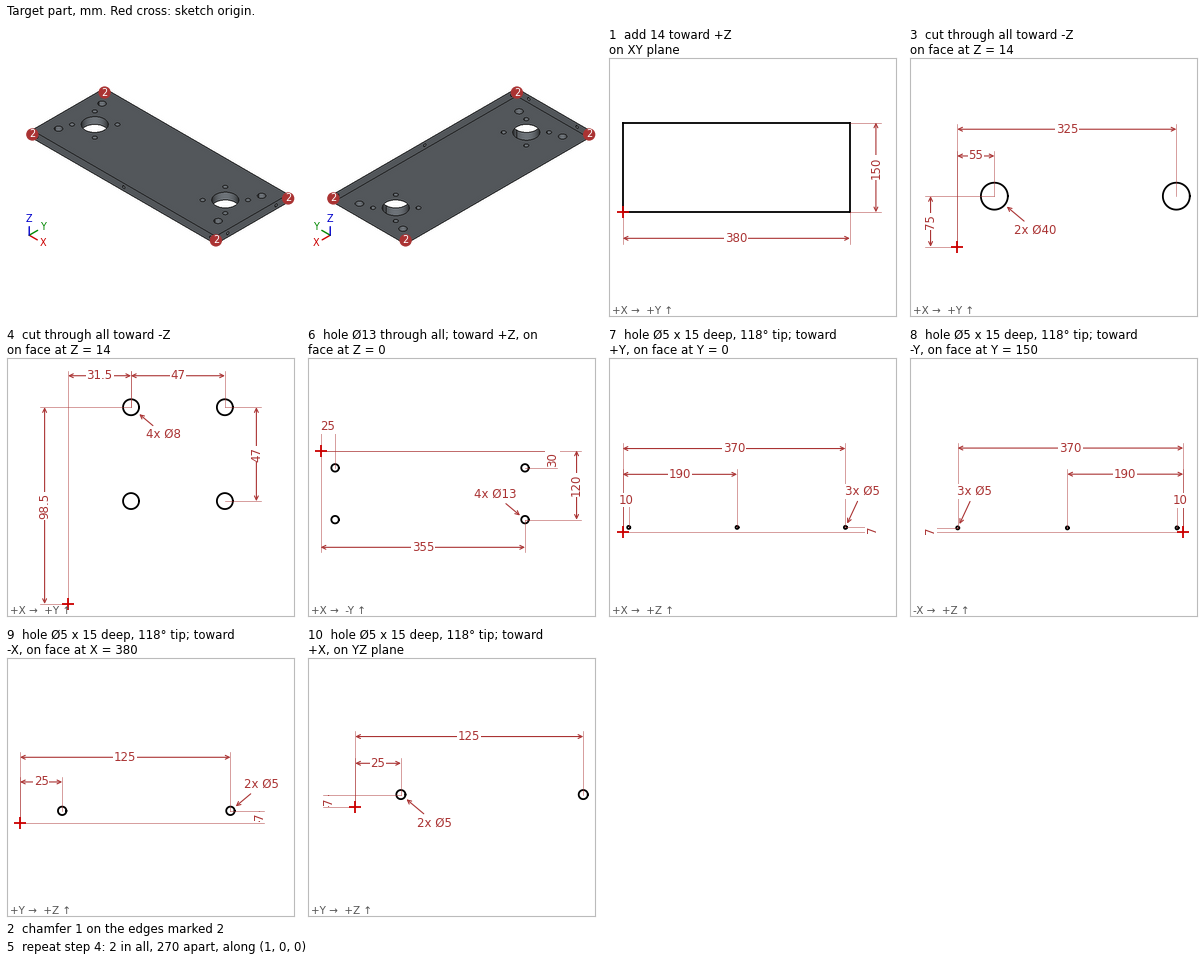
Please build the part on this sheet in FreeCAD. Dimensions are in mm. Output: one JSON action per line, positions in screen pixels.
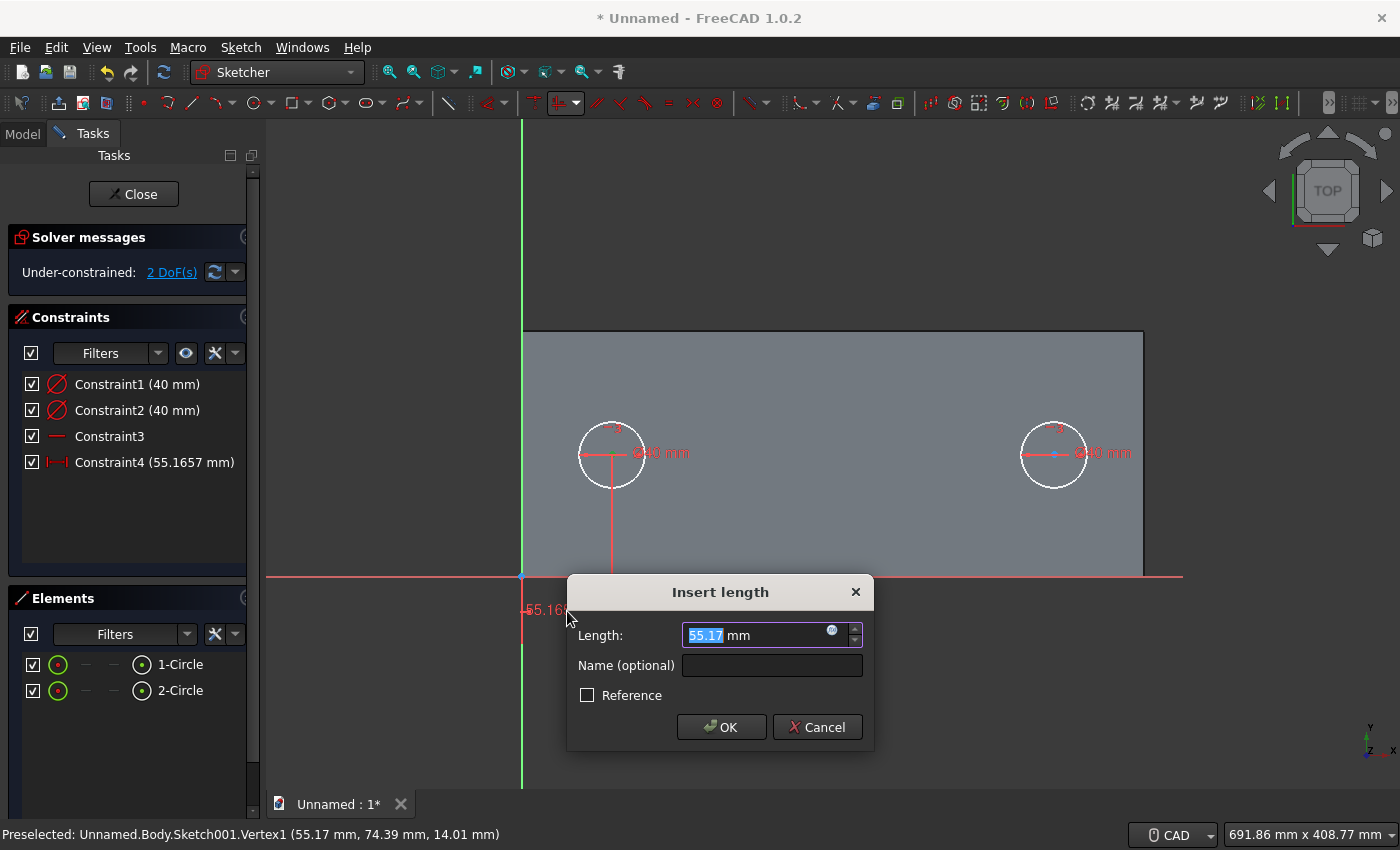
{"action": "type", "text": "55"}
{"action": "key", "text": "Return"}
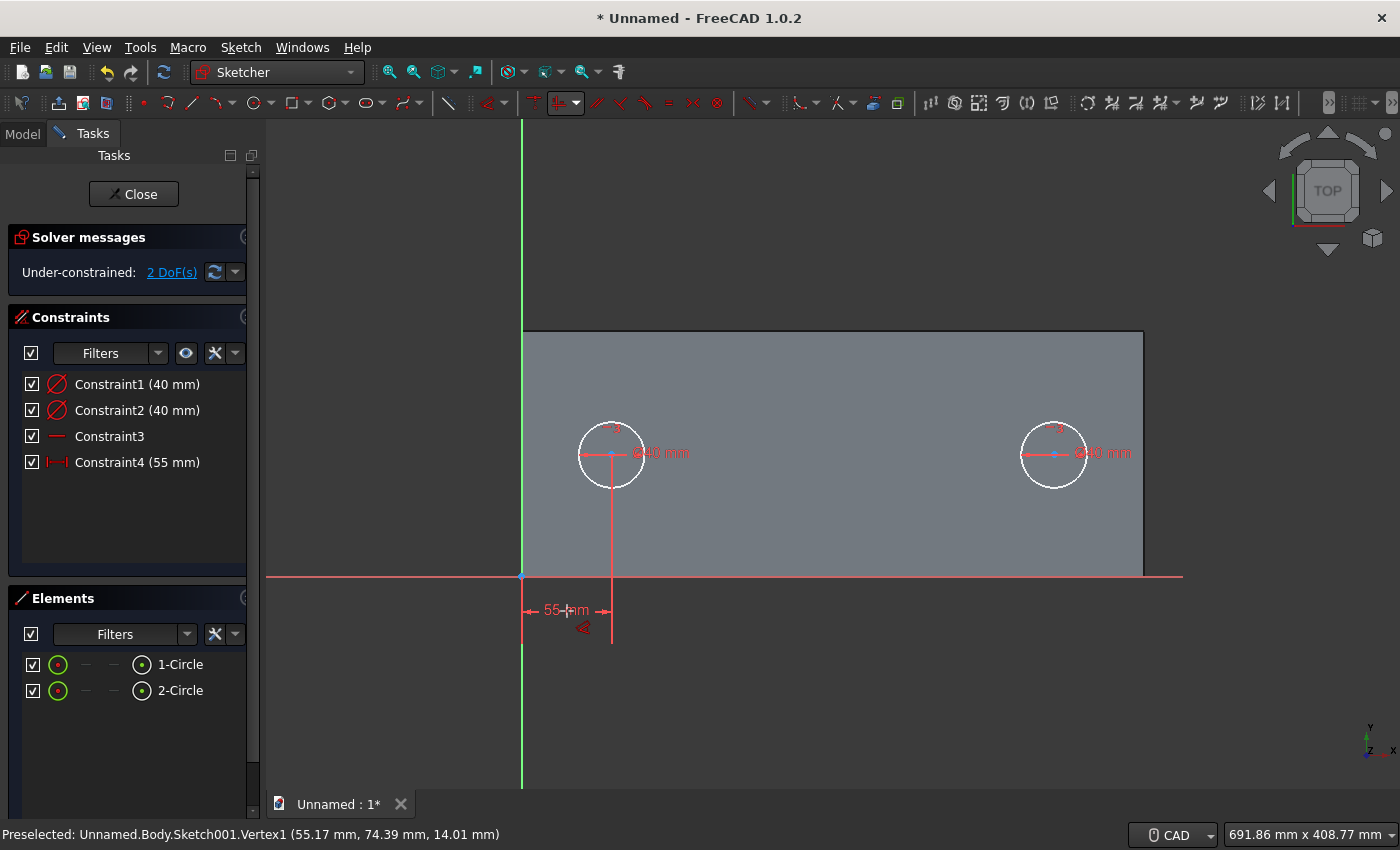
{"action": "left_click", "coordinate": [612, 455]}
{"action": "left_click", "coordinate": [488, 516]}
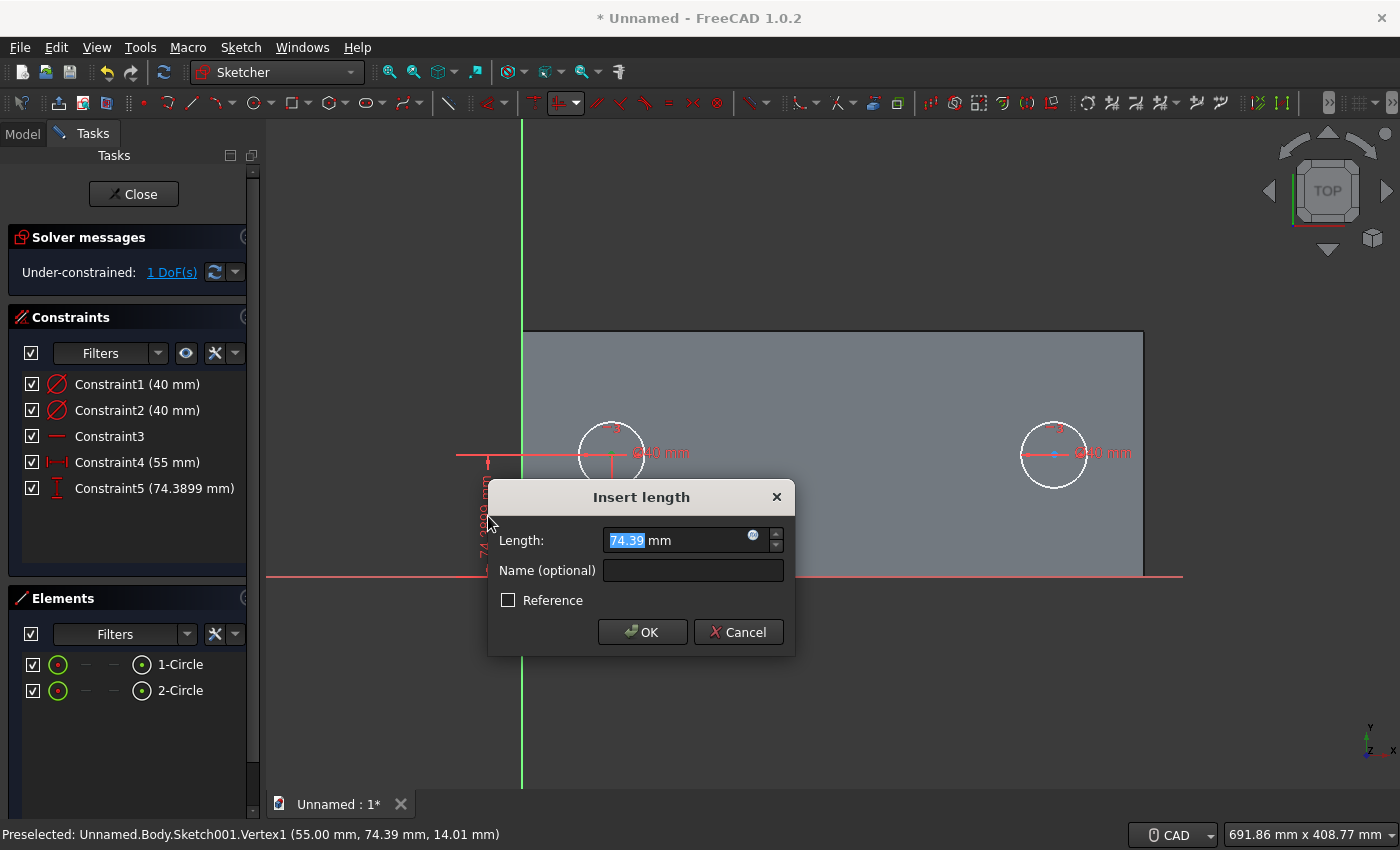
{"action": "type", "text": "75"}
{"action": "key", "text": "Return"}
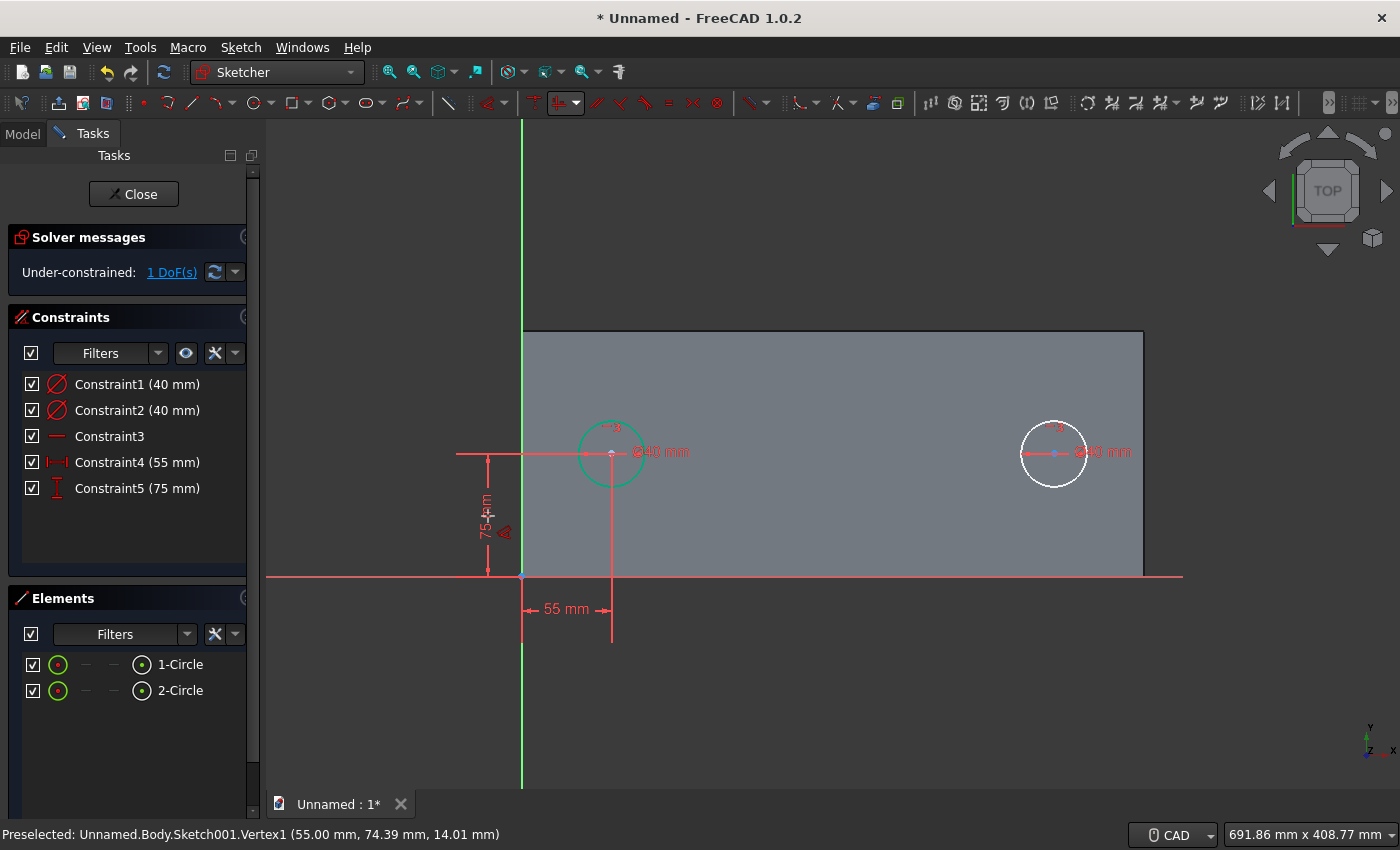
{"action": "left_click", "coordinate": [1054, 454]}
{"action": "left_click", "coordinate": [788, 611]}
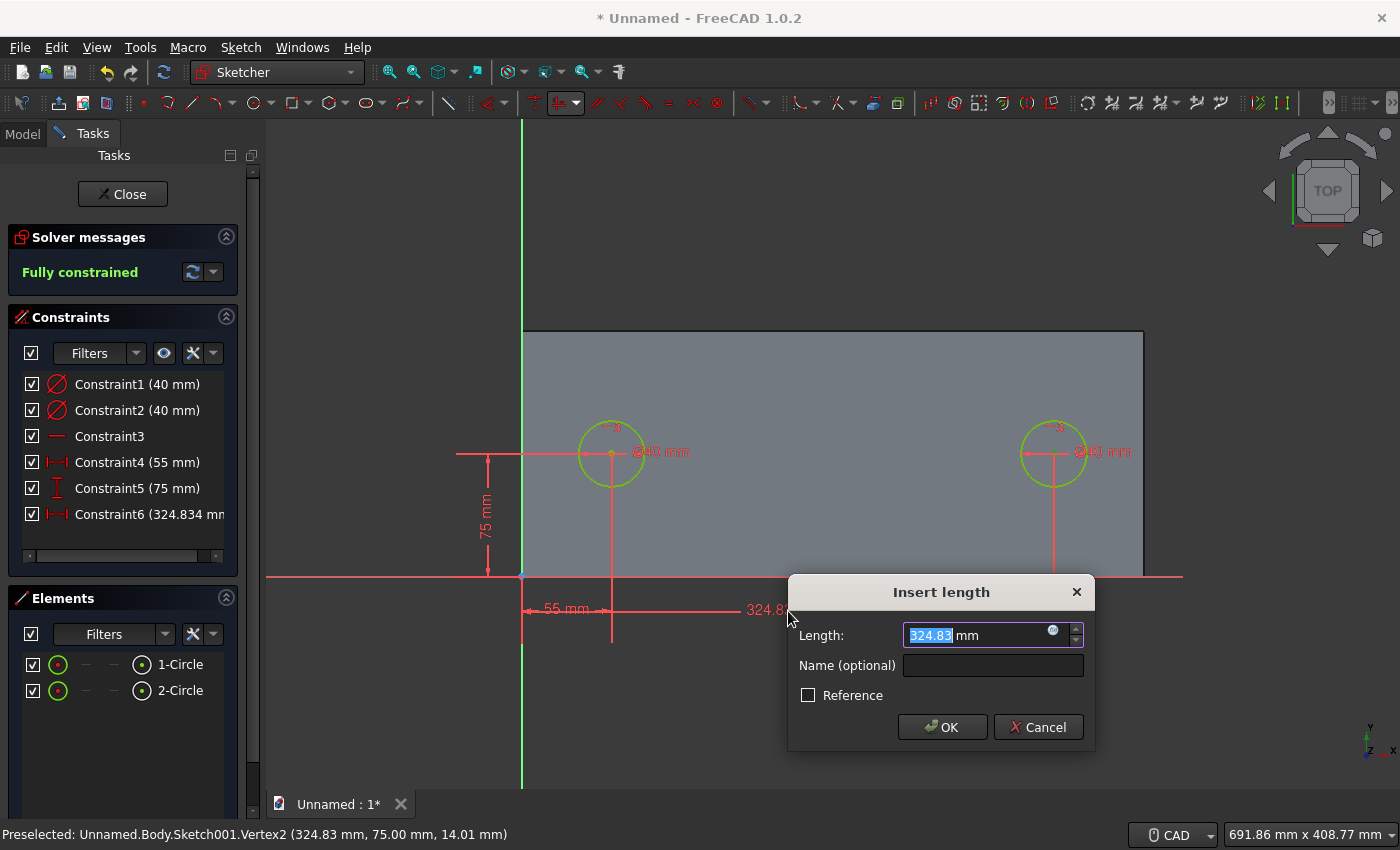
{"action": "type", "text": "325"}
{"action": "key", "text": "Return"}
{"action": "key", "text": "Escape"}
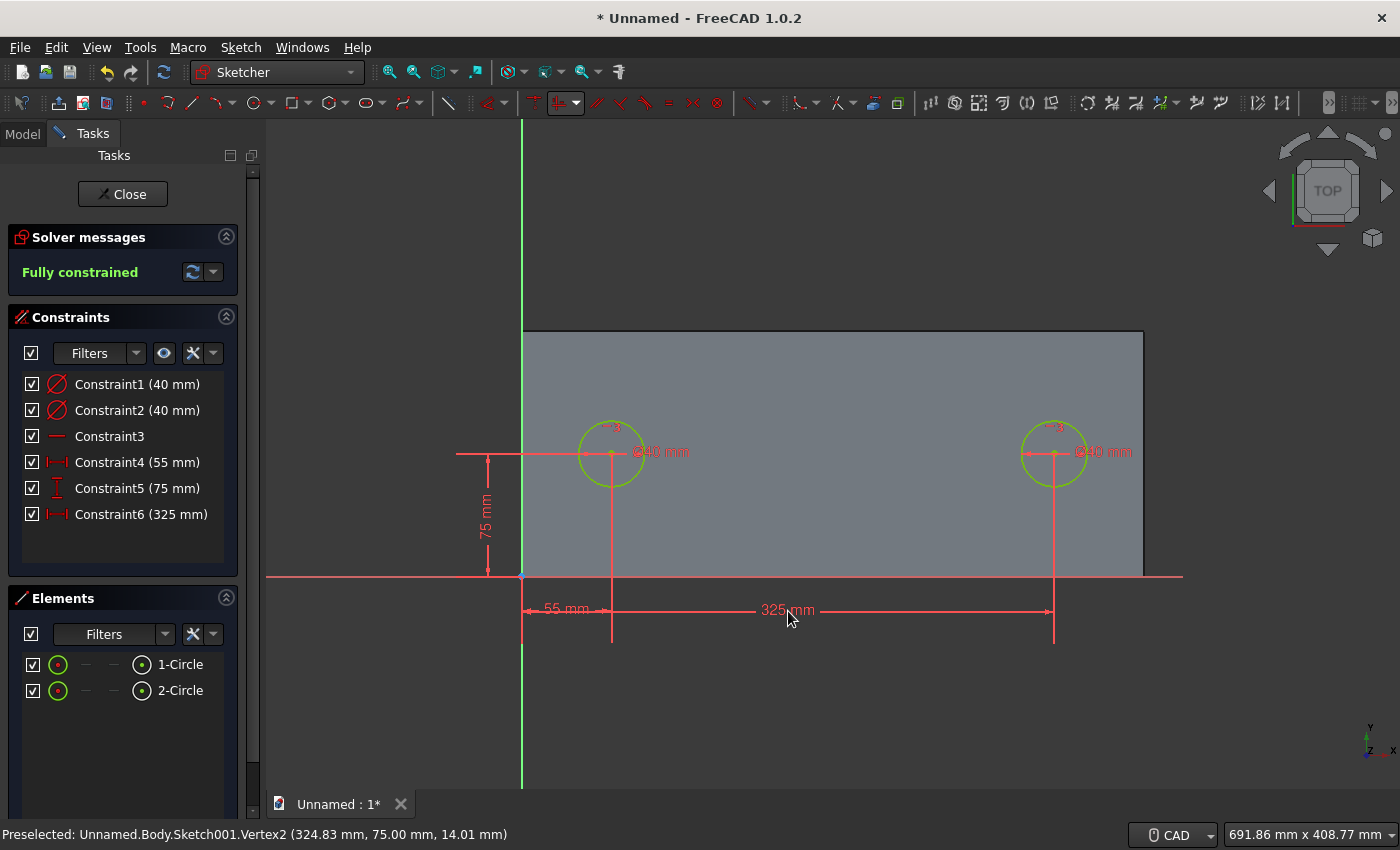
{"action": "left_click", "coordinate": [123, 194]}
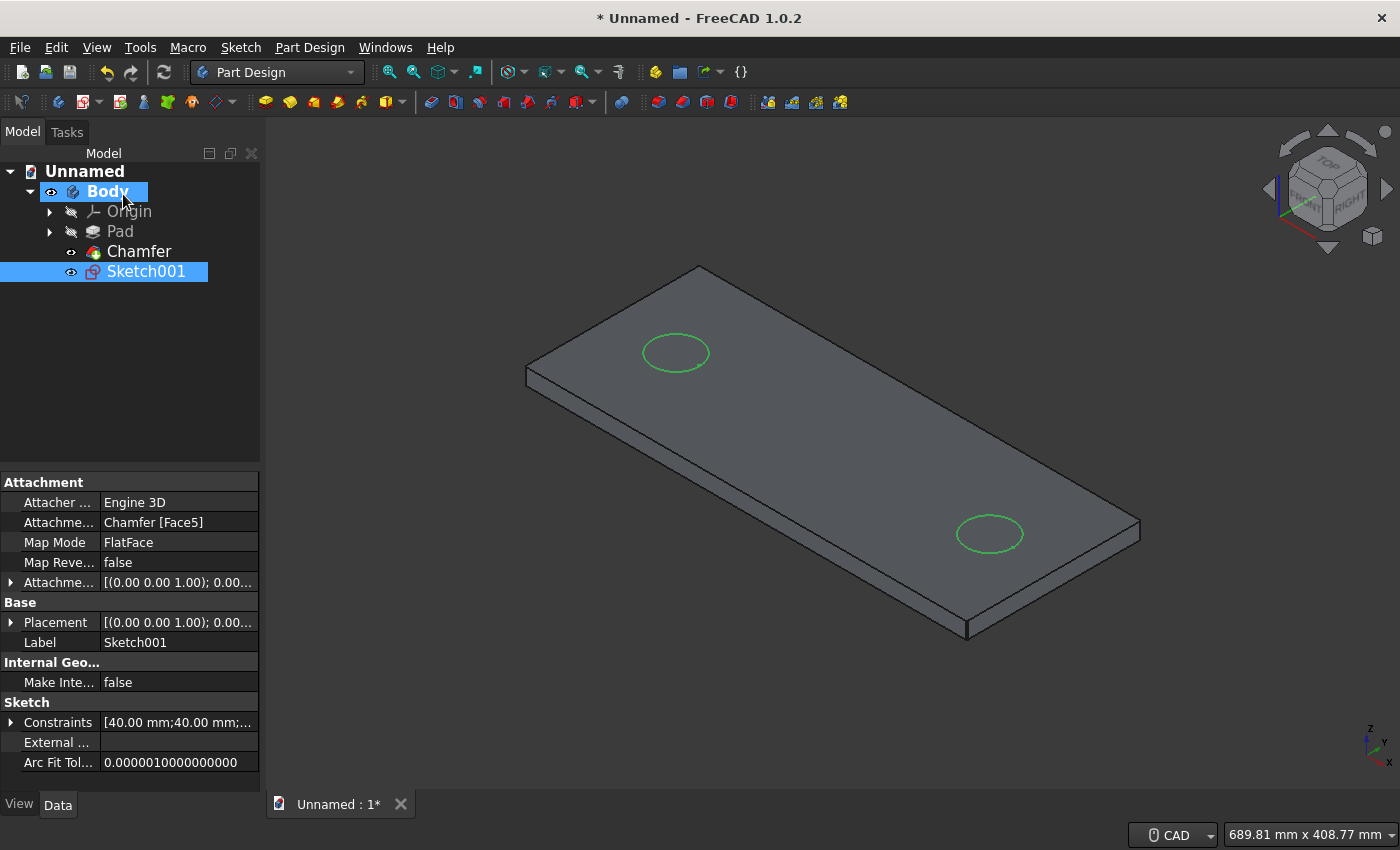
{"action": "left_click", "coordinate": [432, 102]}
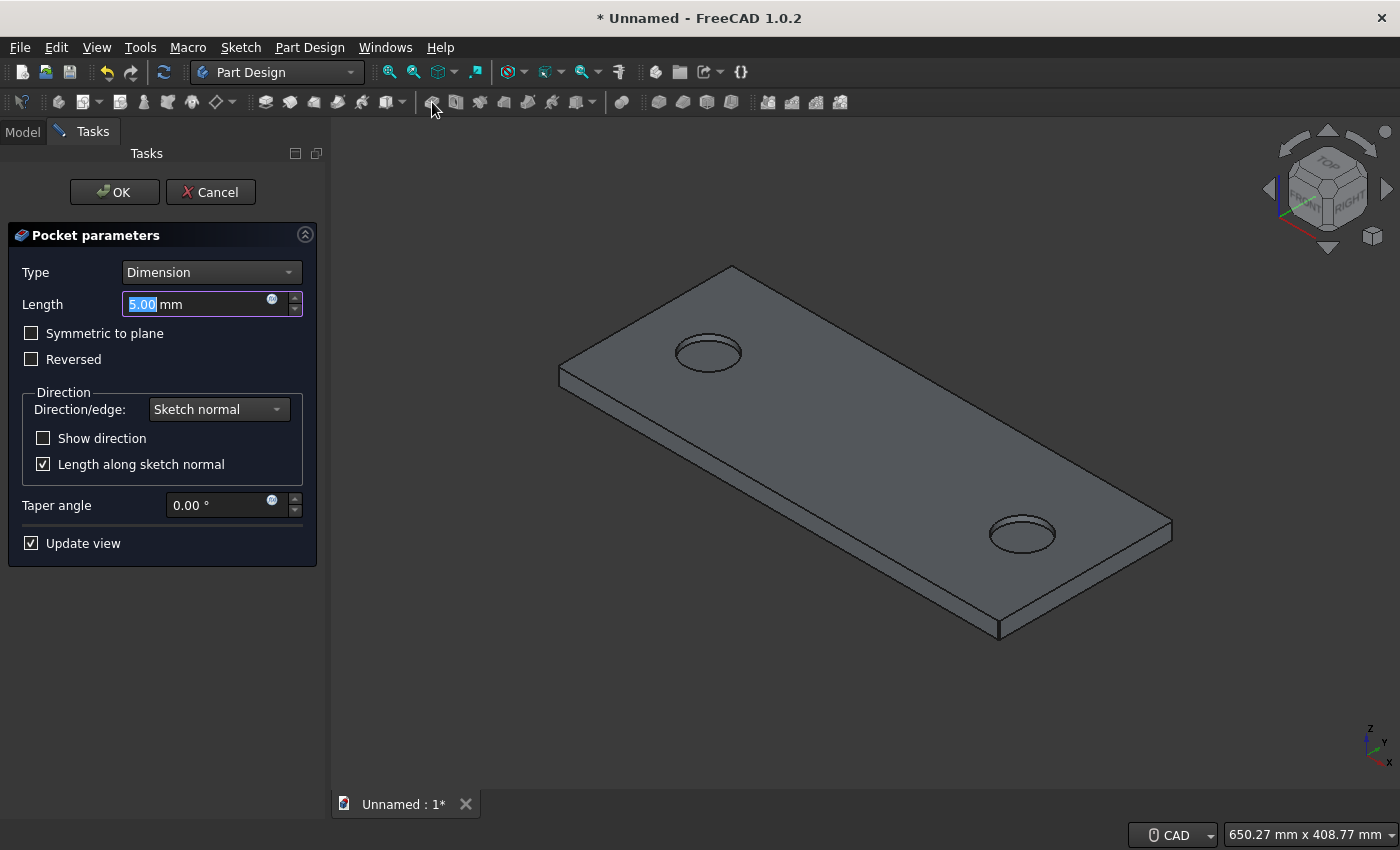
{"action": "left_click", "coordinate": [212, 272]}